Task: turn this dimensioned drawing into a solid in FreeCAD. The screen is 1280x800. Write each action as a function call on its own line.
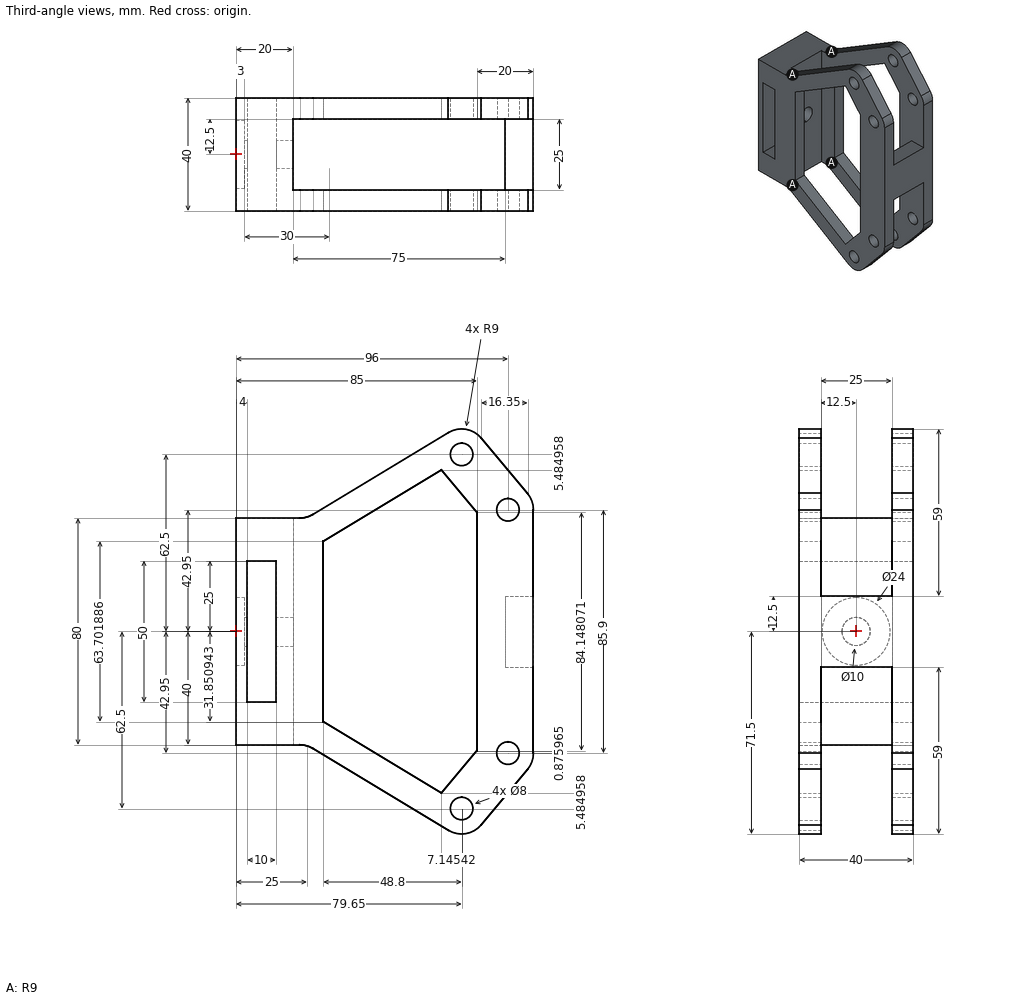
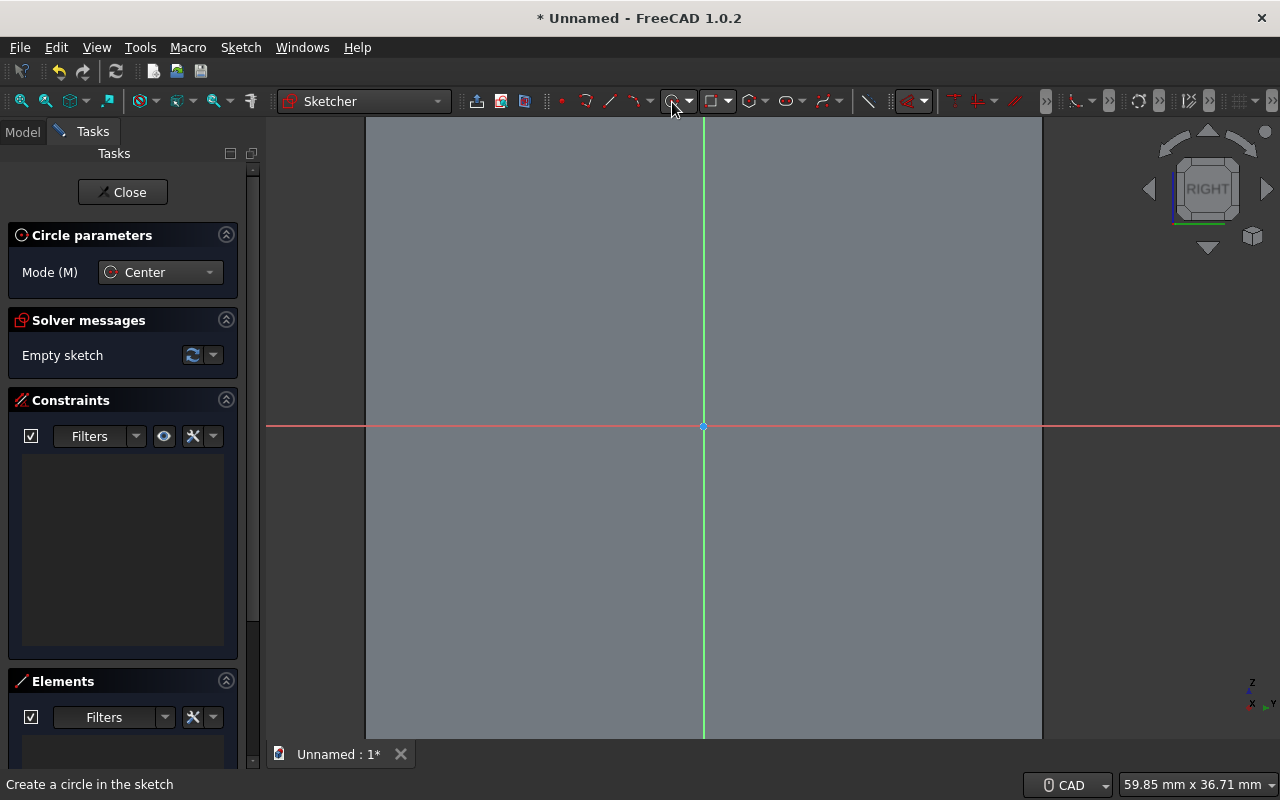
click(704, 426)
move(848, 282)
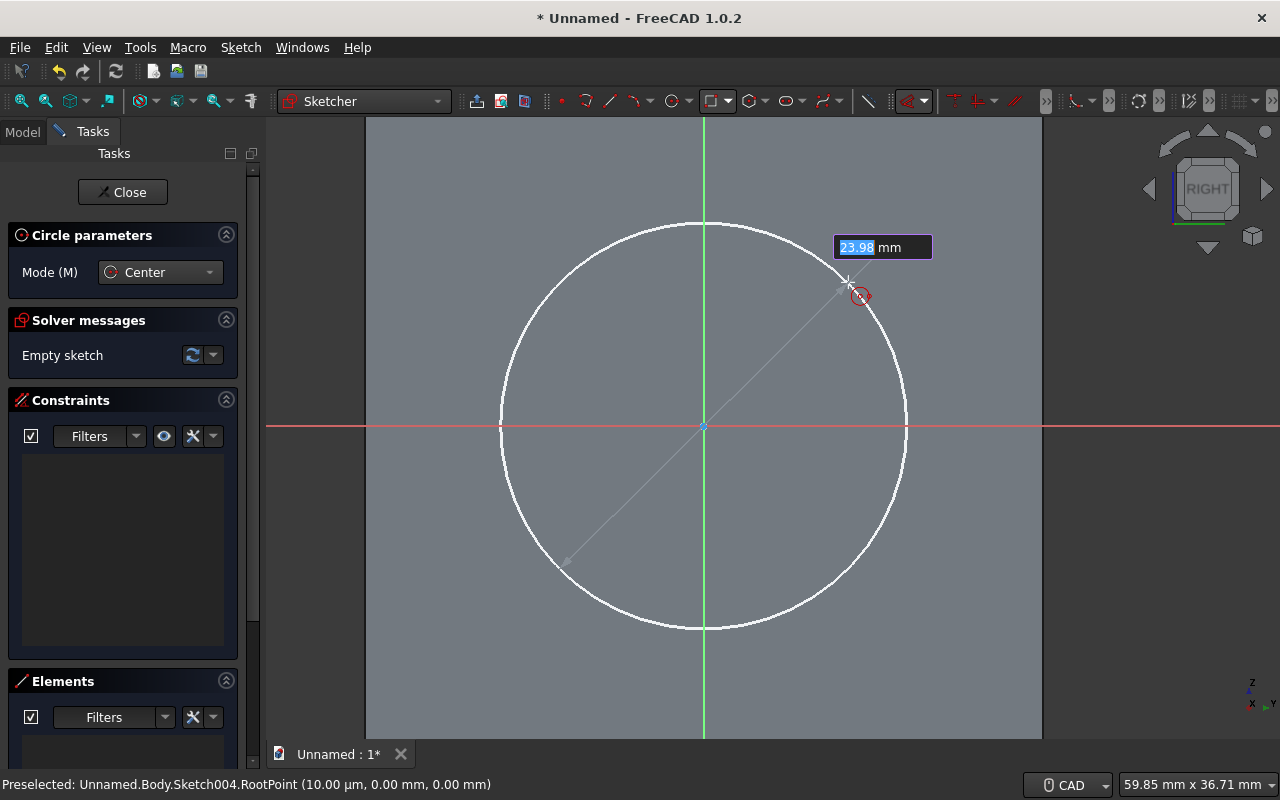
text(24)
key(Return)
key(Escape)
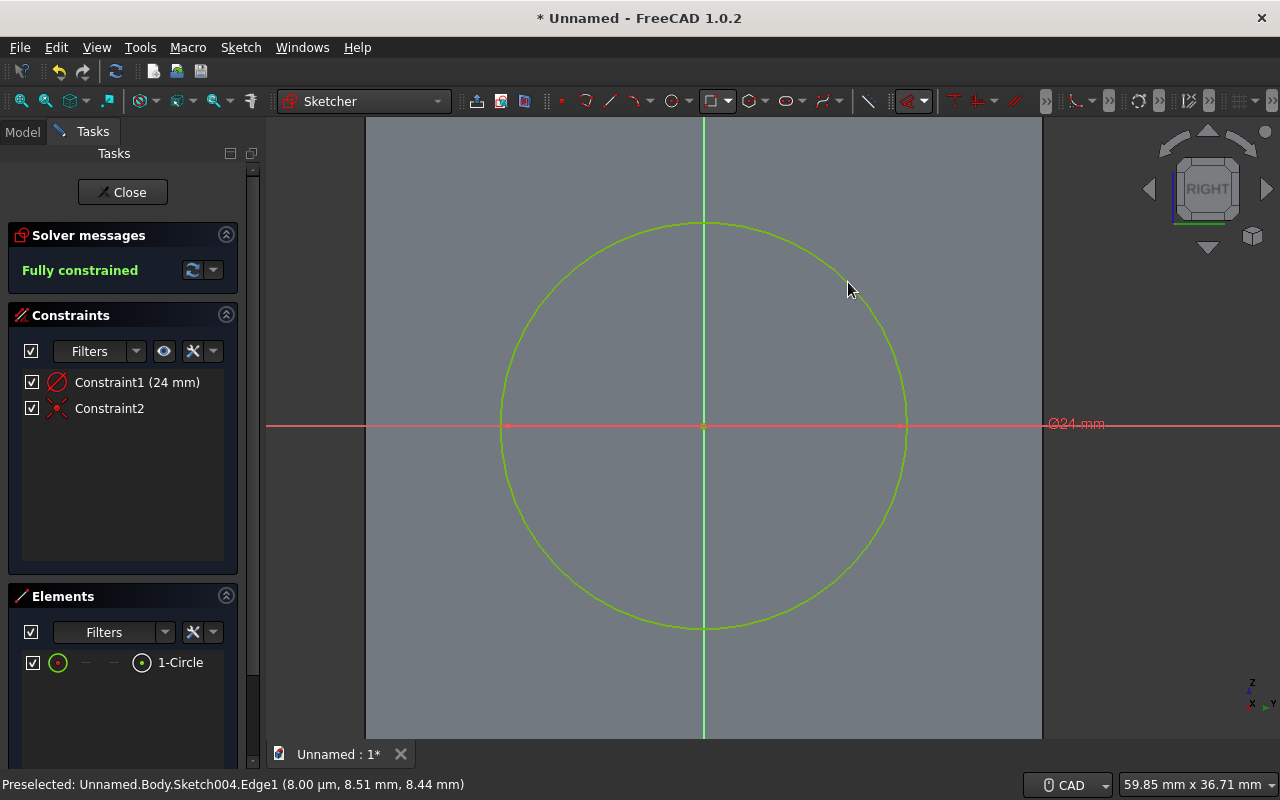
click(123, 192)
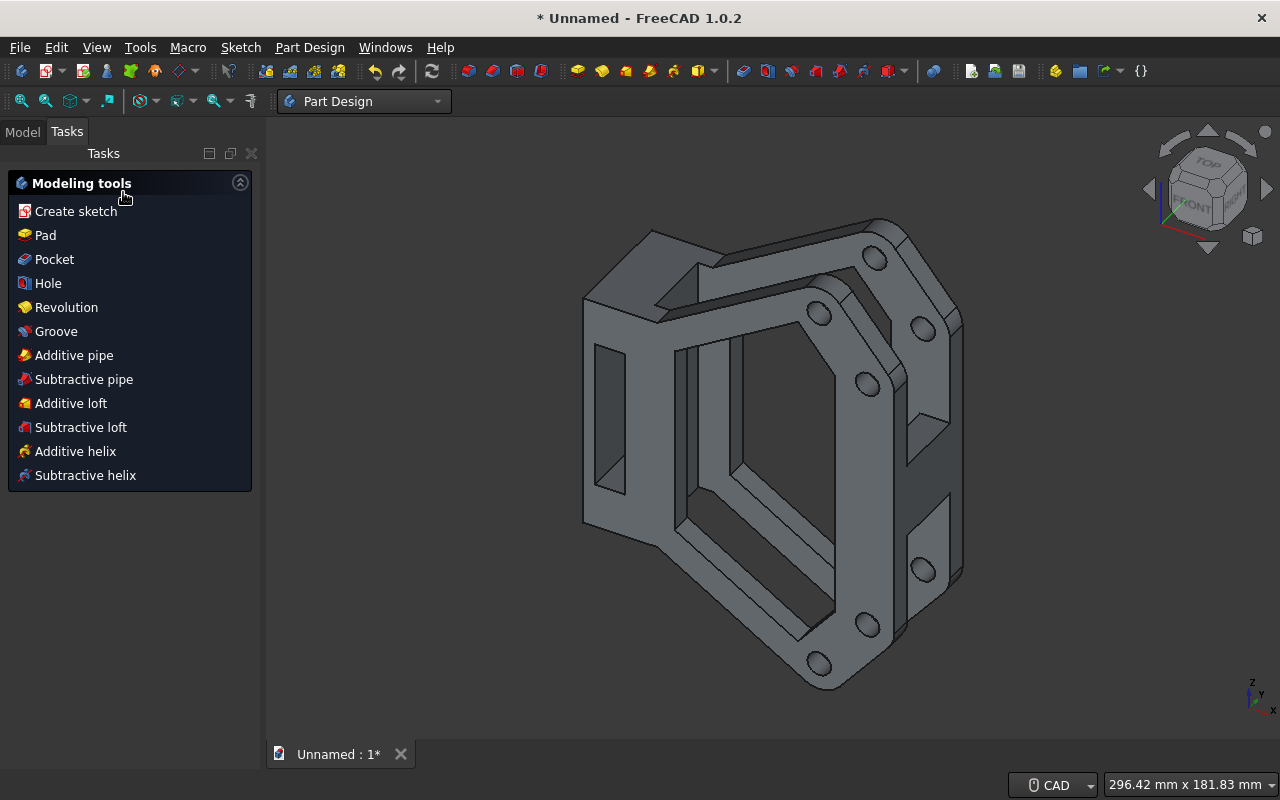
click(744, 72)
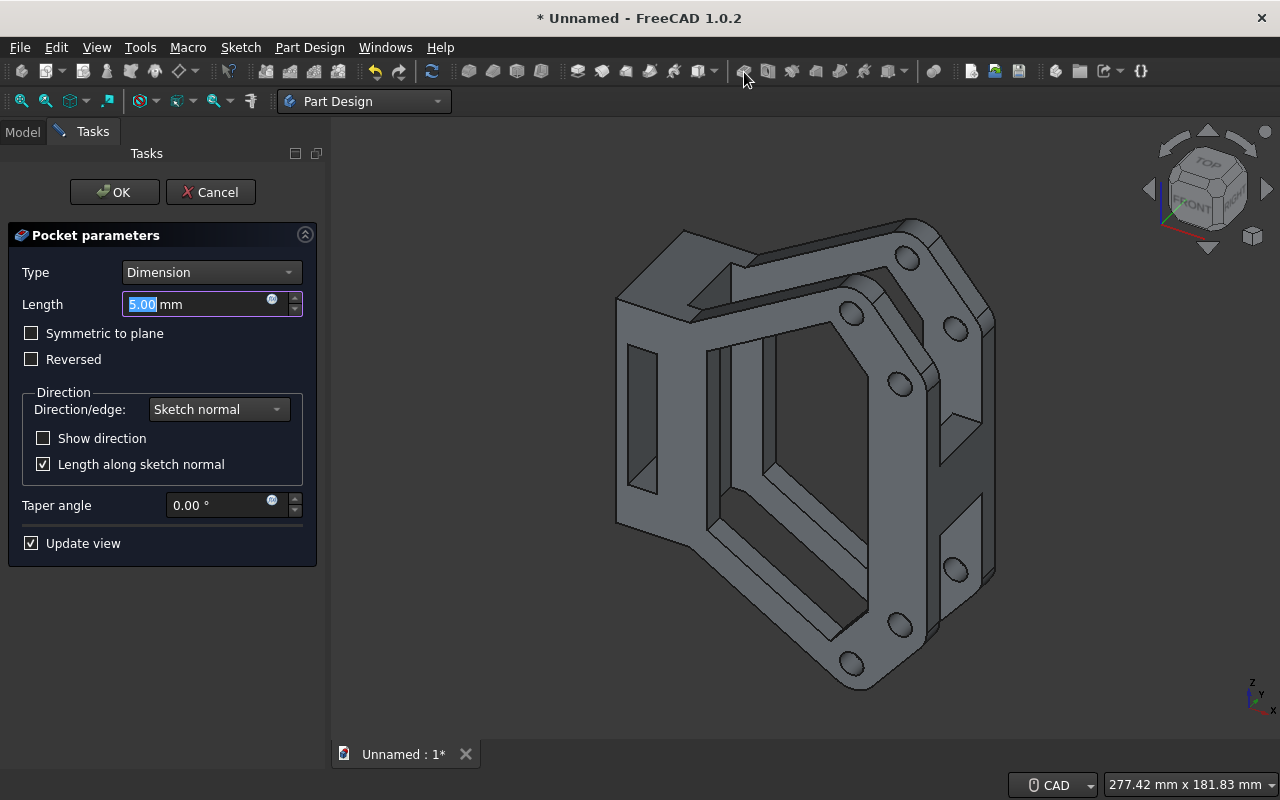
text(3)
key(Tab)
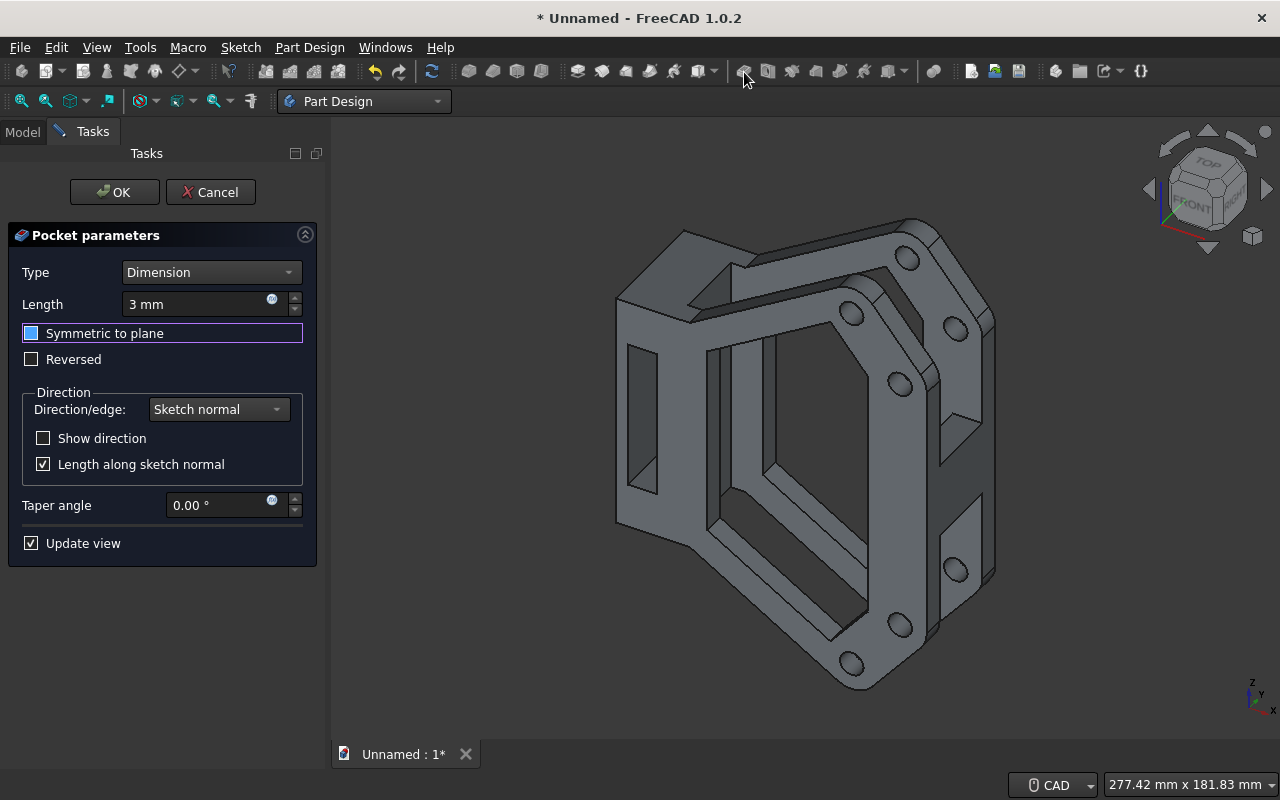
click(30, 359)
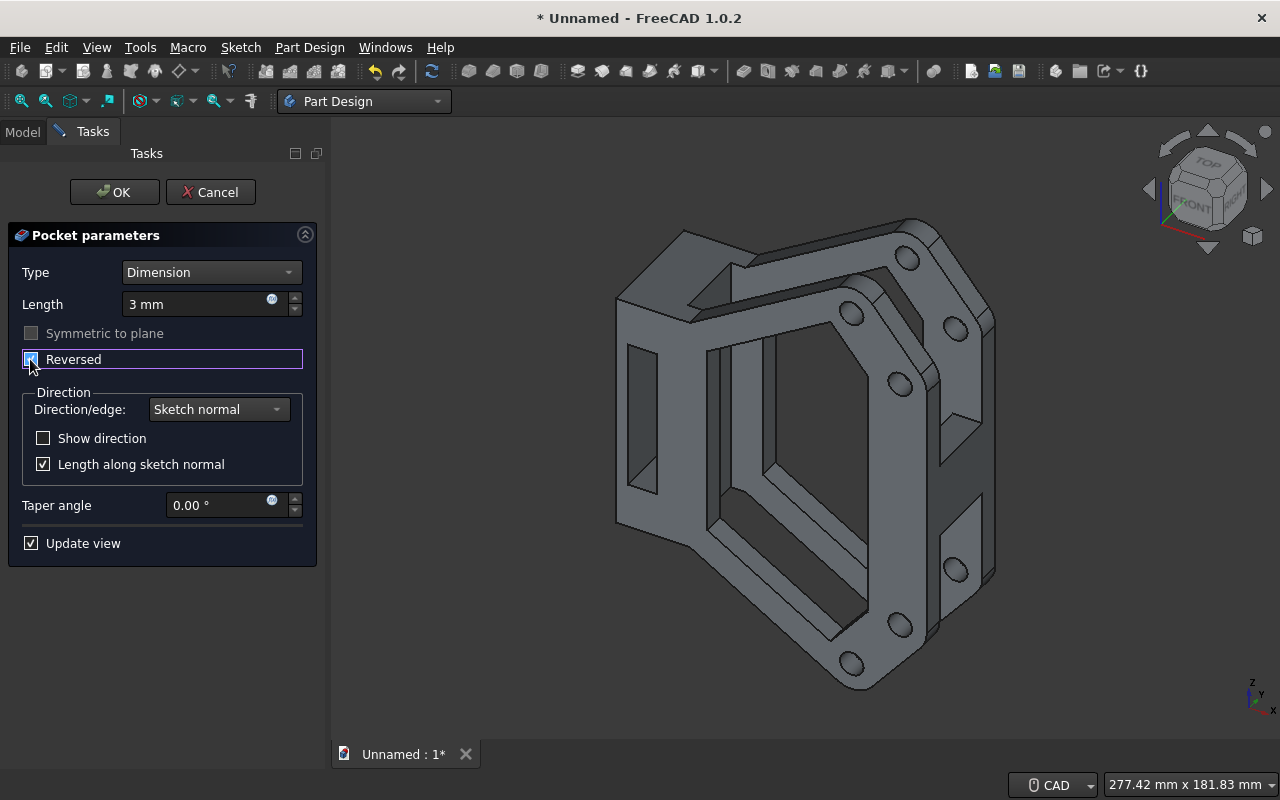
click(115, 192)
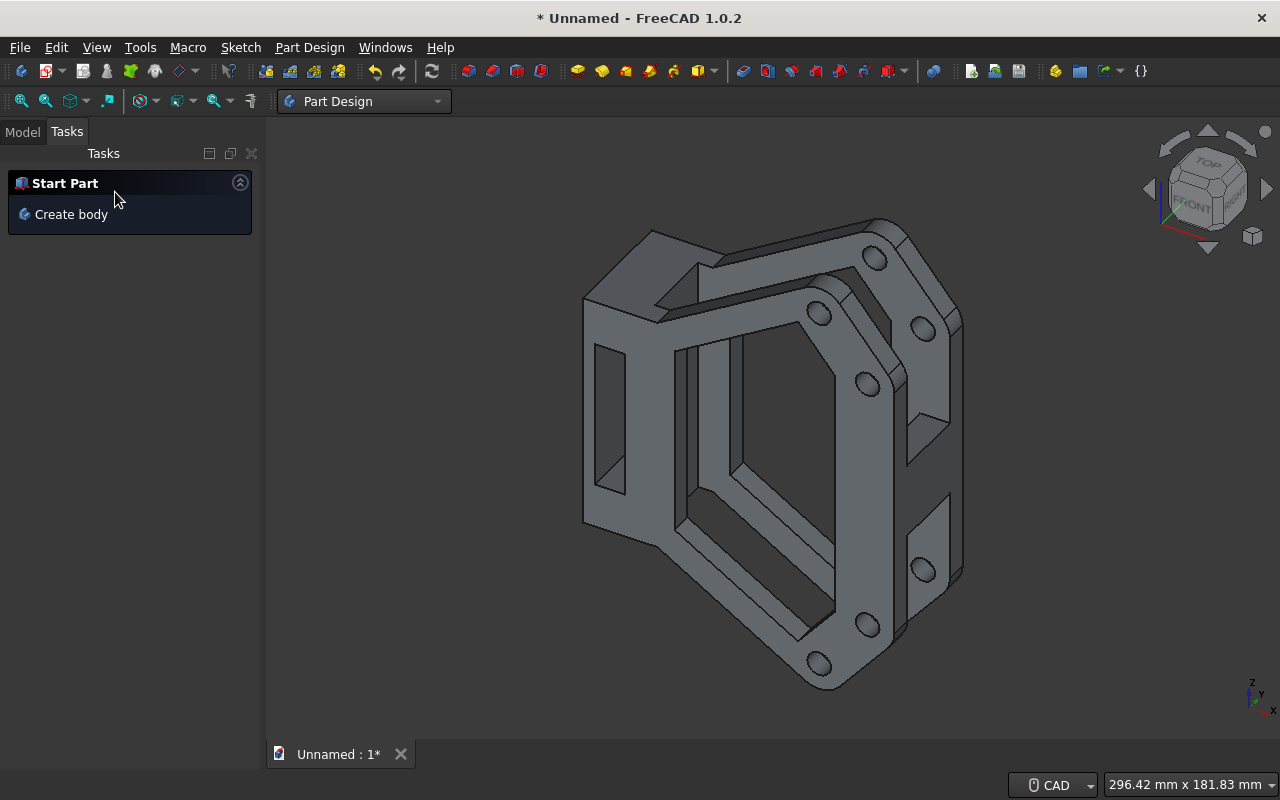
key(6)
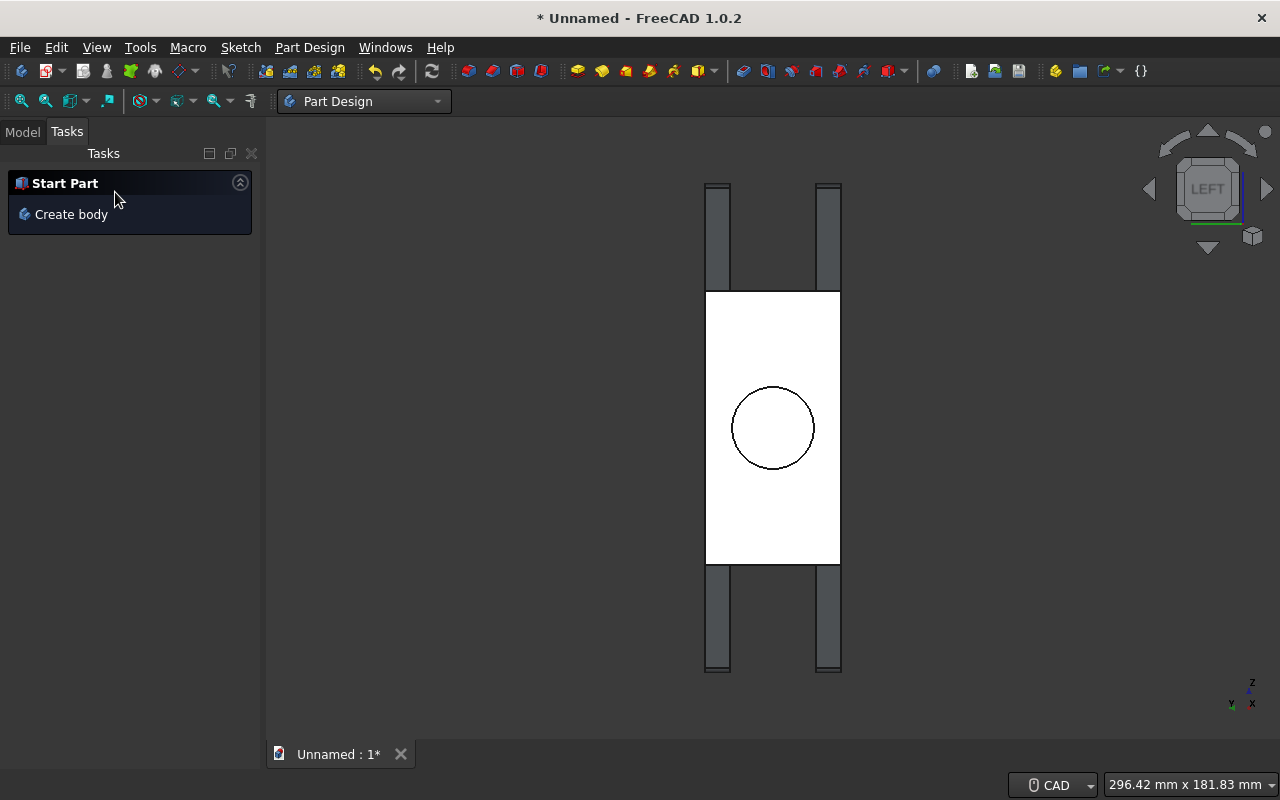
click(773, 427)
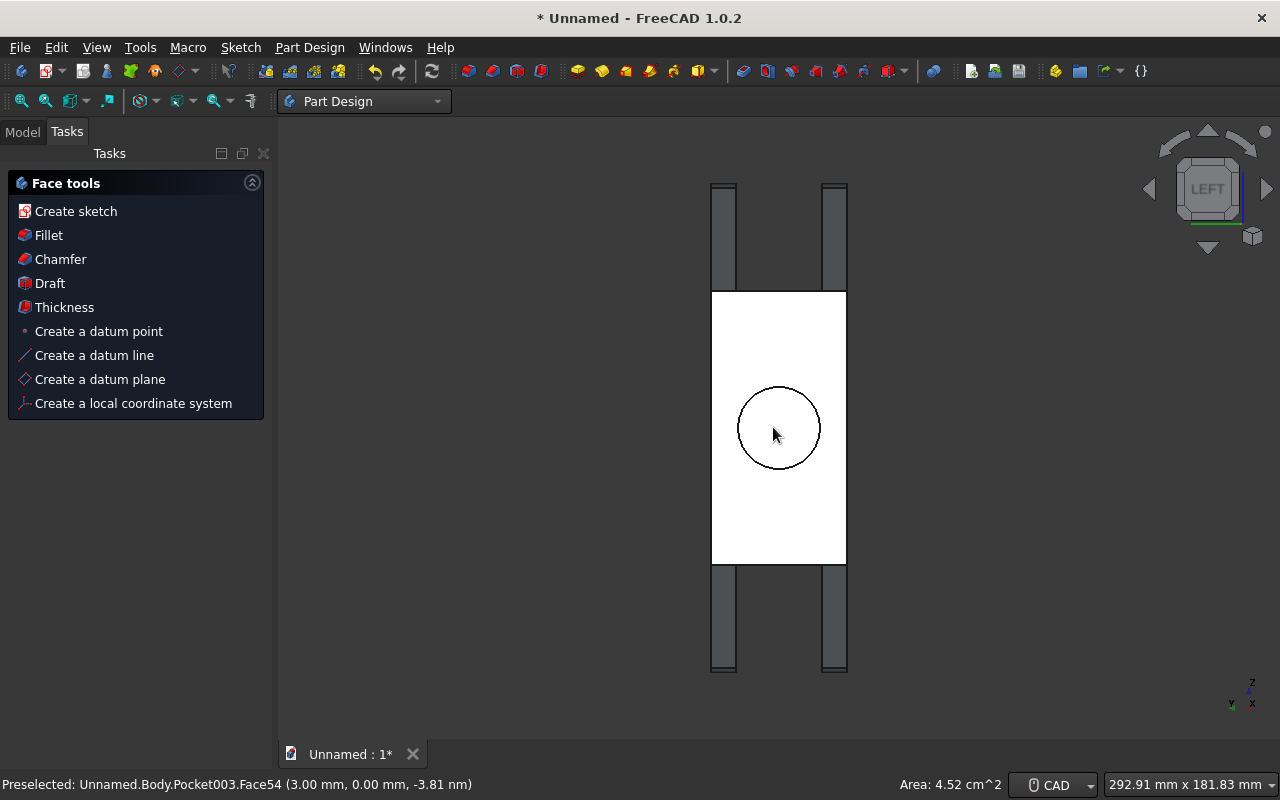
click(46, 72)